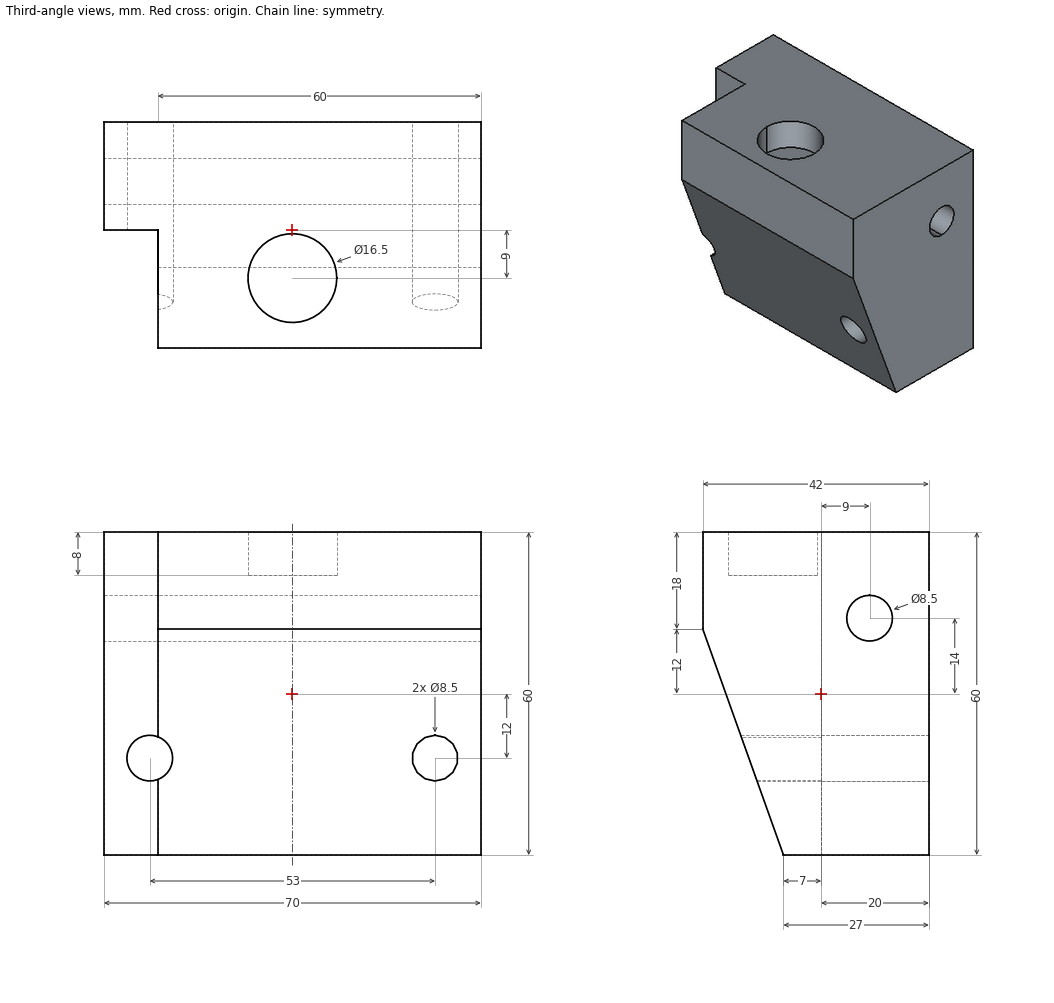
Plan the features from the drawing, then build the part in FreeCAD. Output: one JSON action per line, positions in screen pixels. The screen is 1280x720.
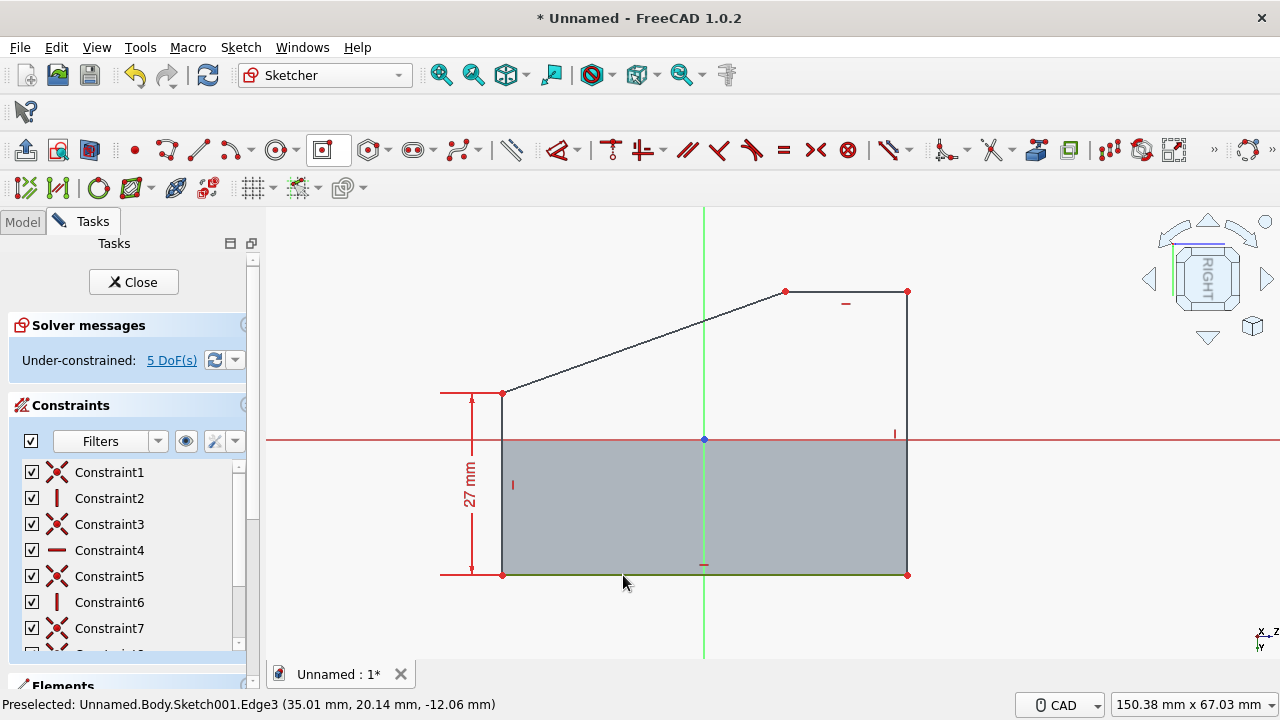
{"action": "left_click", "coordinate": [580, 150]}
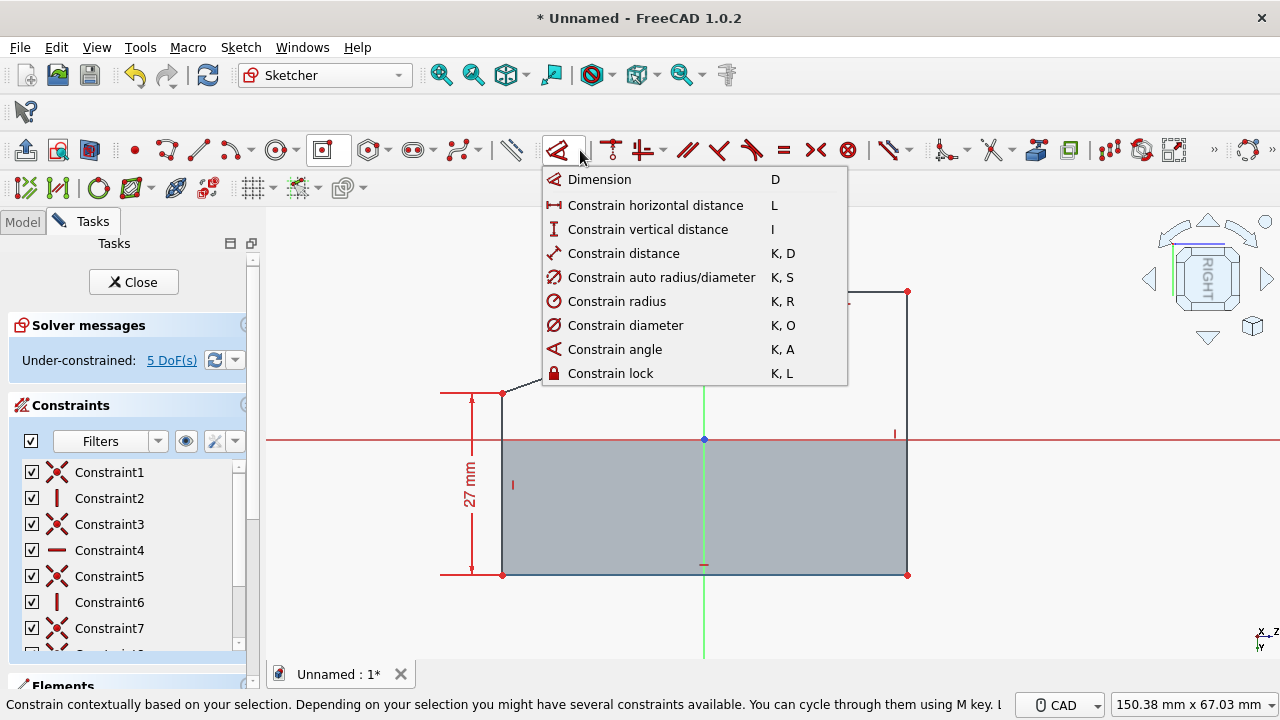
{"action": "left_click", "coordinate": [695, 205]}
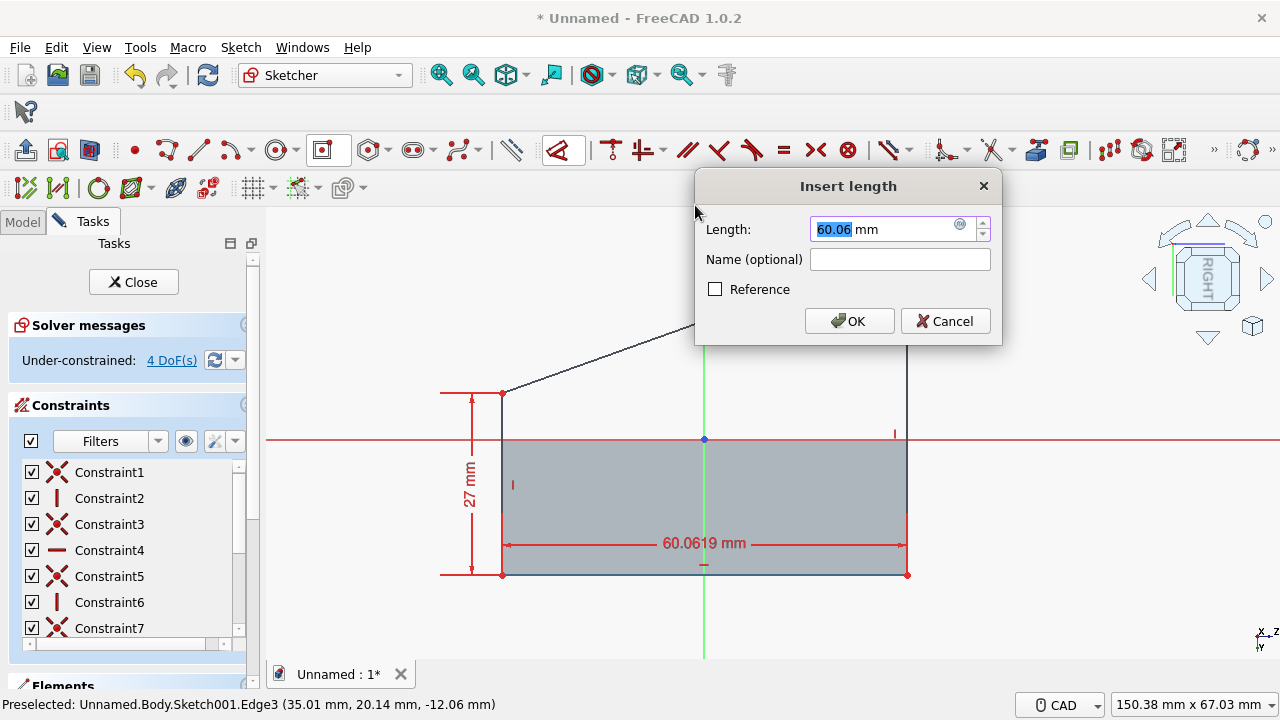
{"action": "type", "text": "60"}
{"action": "key", "text": "Return"}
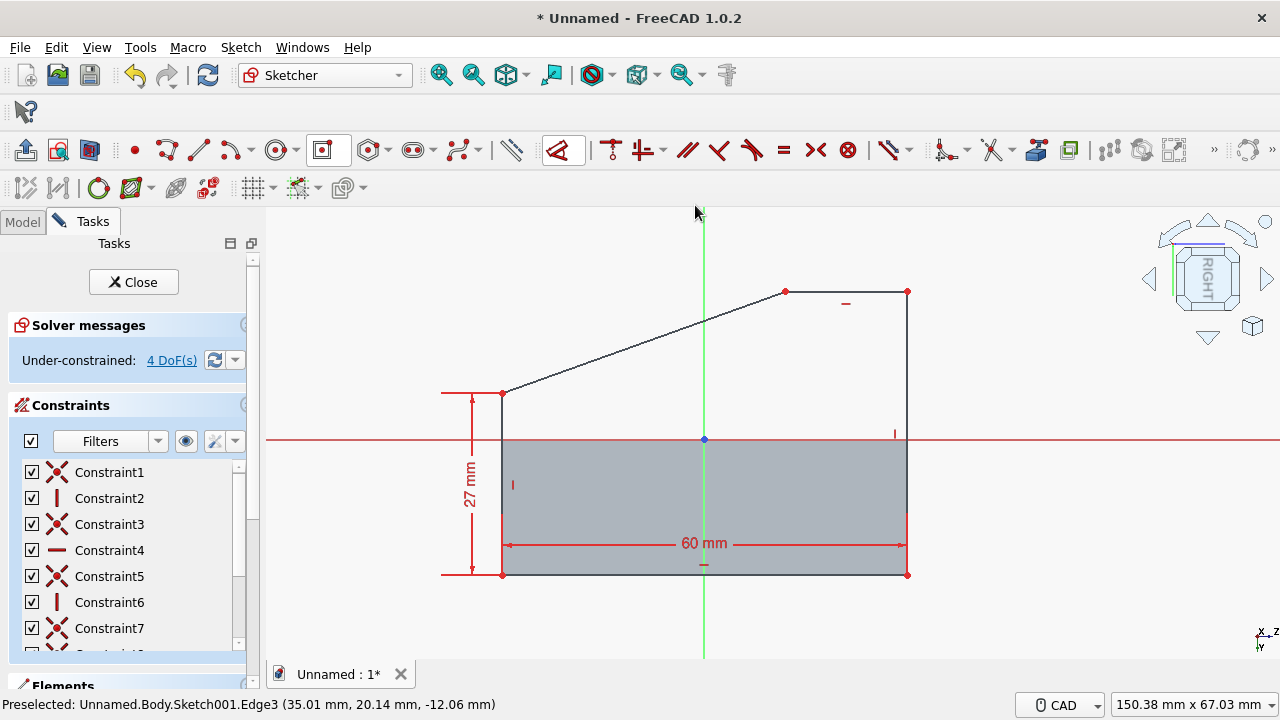
{"action": "left_click", "coordinate": [907, 490]}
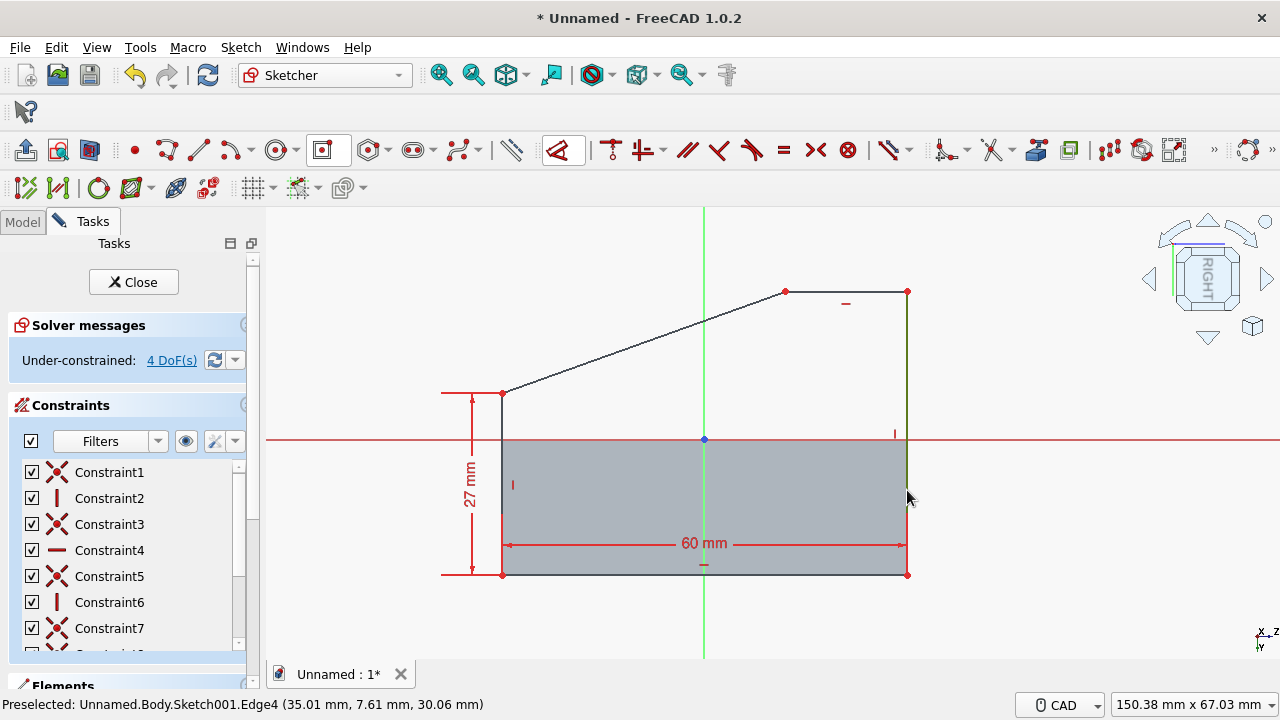
{"action": "key", "text": "i"}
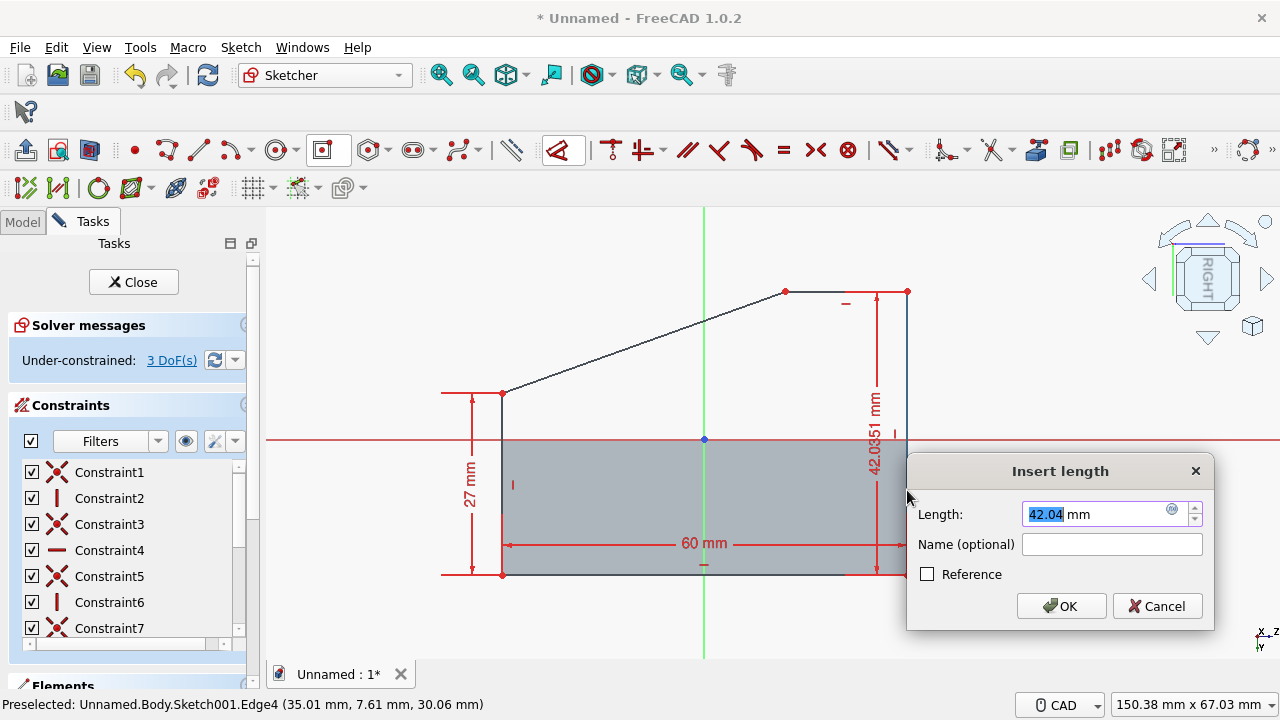
{"action": "type", "text": "42"}
{"action": "key", "text": "Return"}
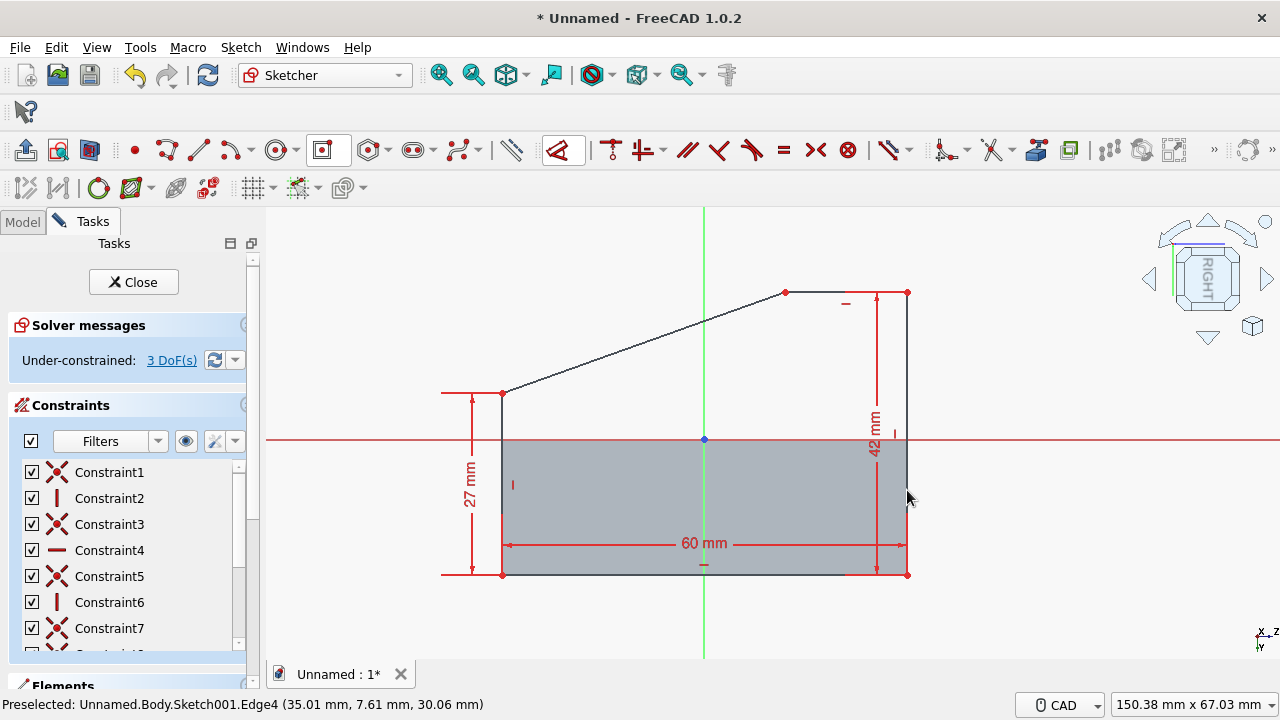
{"action": "left_click", "coordinate": [870, 292]}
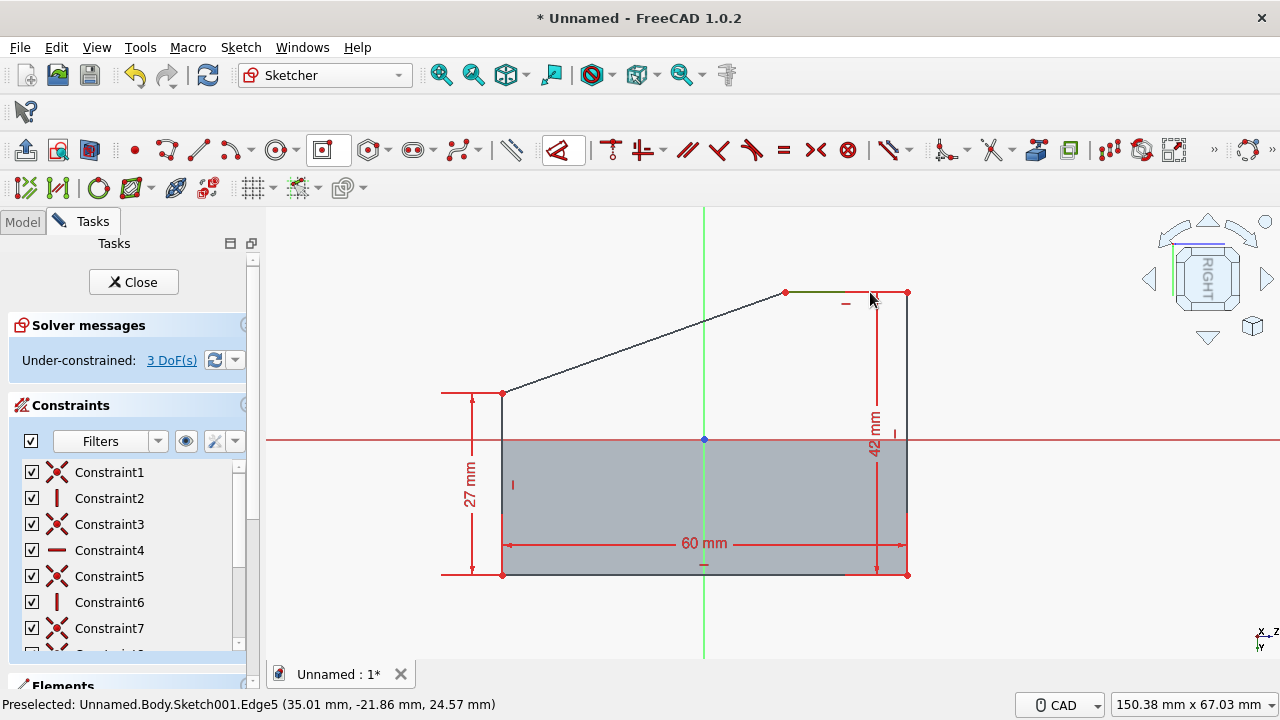
{"action": "left_click", "coordinate": [580, 150]}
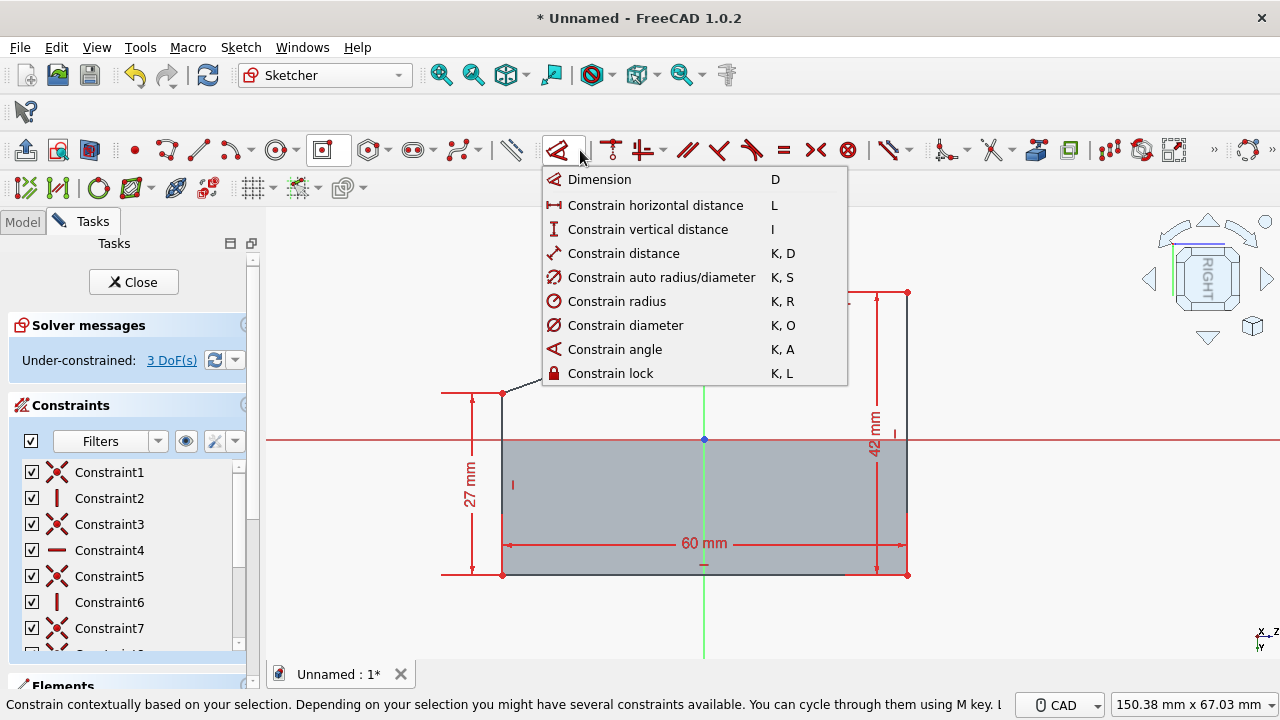
{"action": "left_click", "coordinate": [695, 205]}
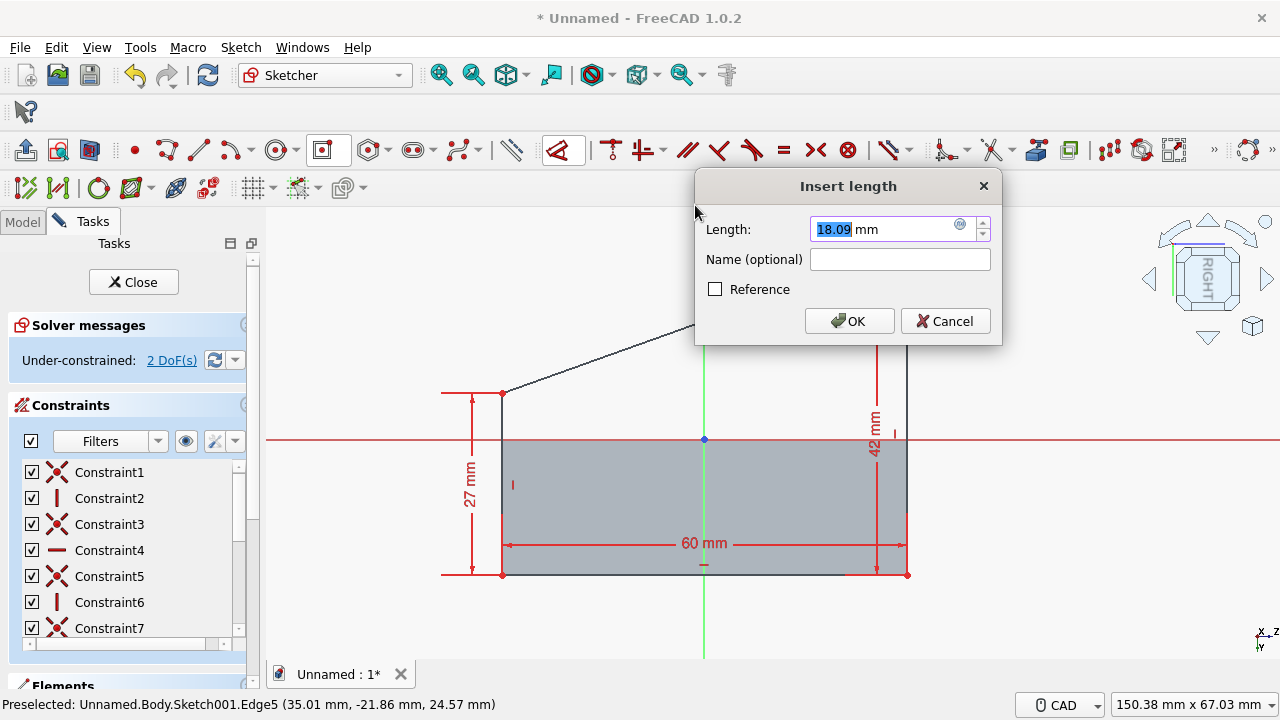
{"action": "type", "text": "18"}
{"action": "key", "text": "Return"}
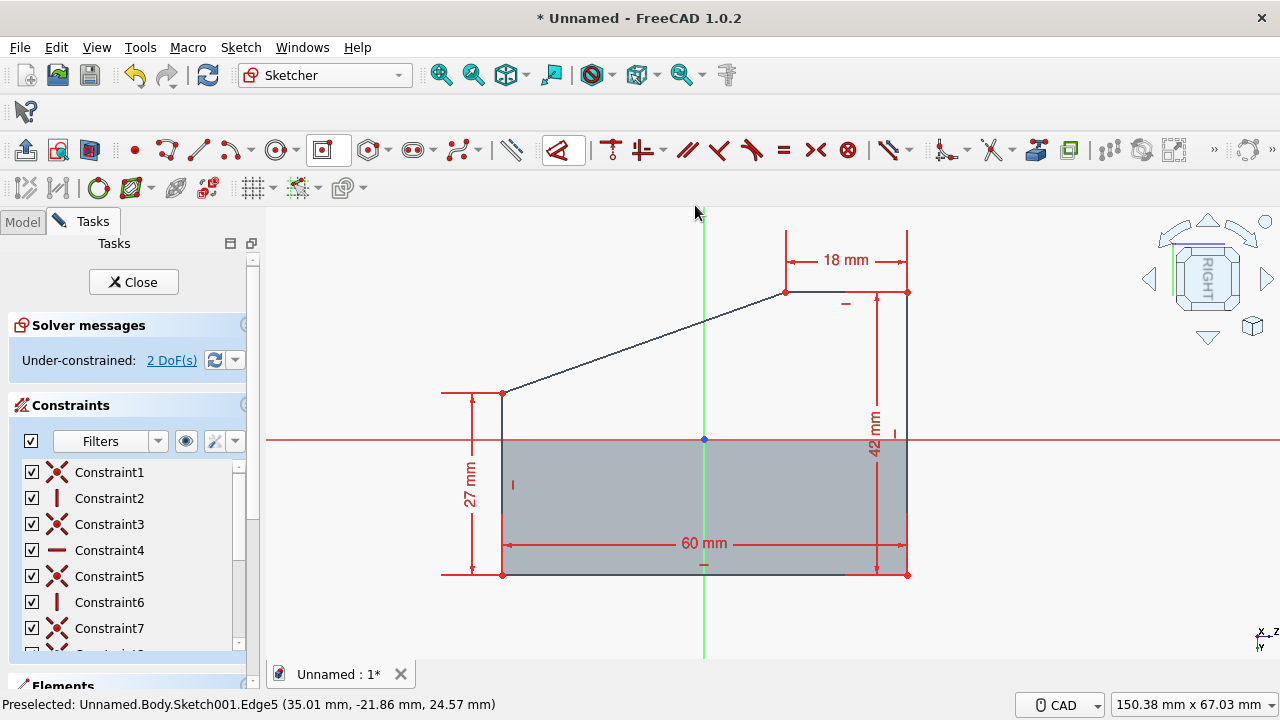
{"action": "left_click", "coordinate": [502, 393]}